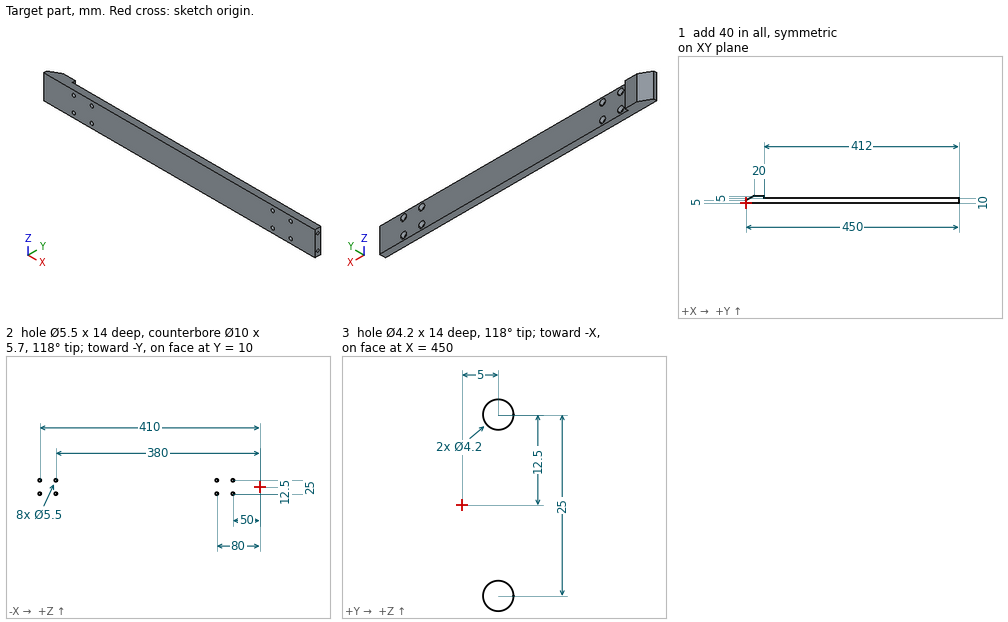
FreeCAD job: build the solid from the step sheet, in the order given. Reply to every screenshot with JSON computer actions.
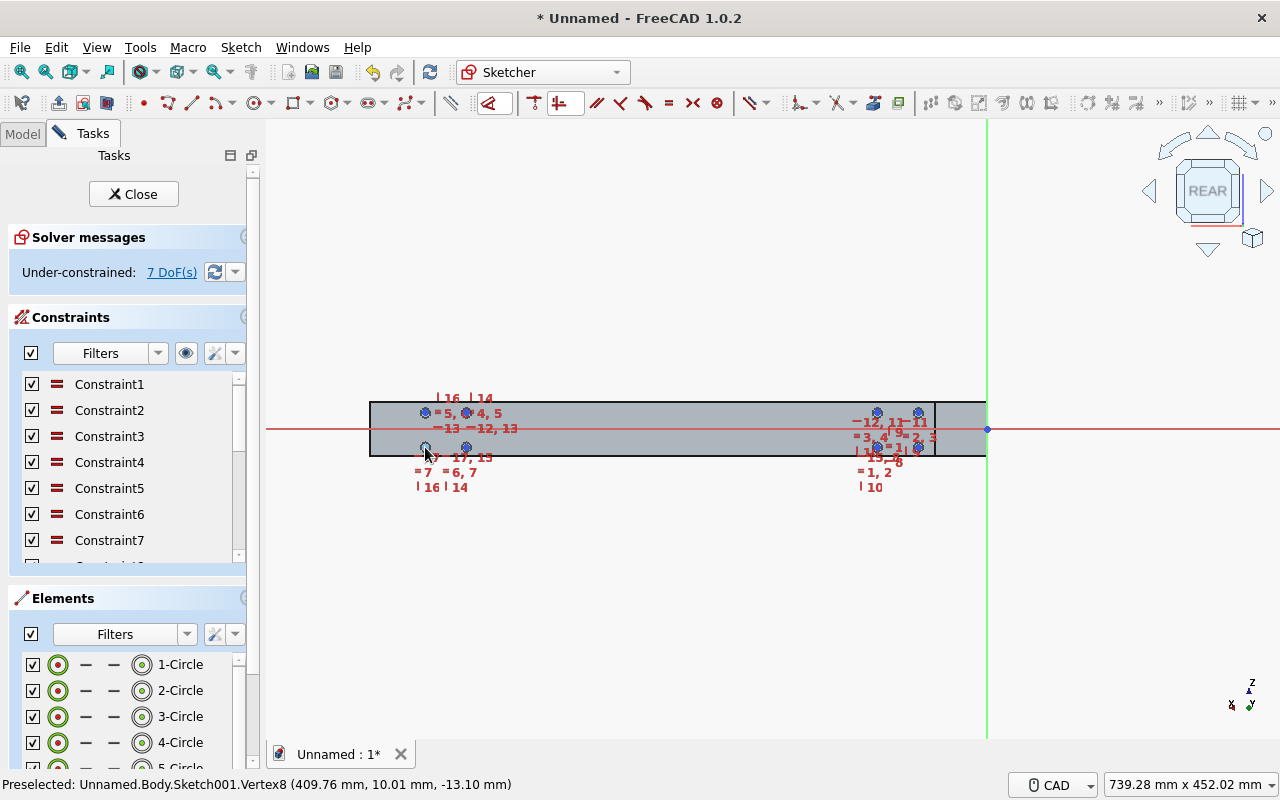
{"action": "scroll", "coordinate": [922, 444], "scroll_direction": "up", "scroll_amount": 9}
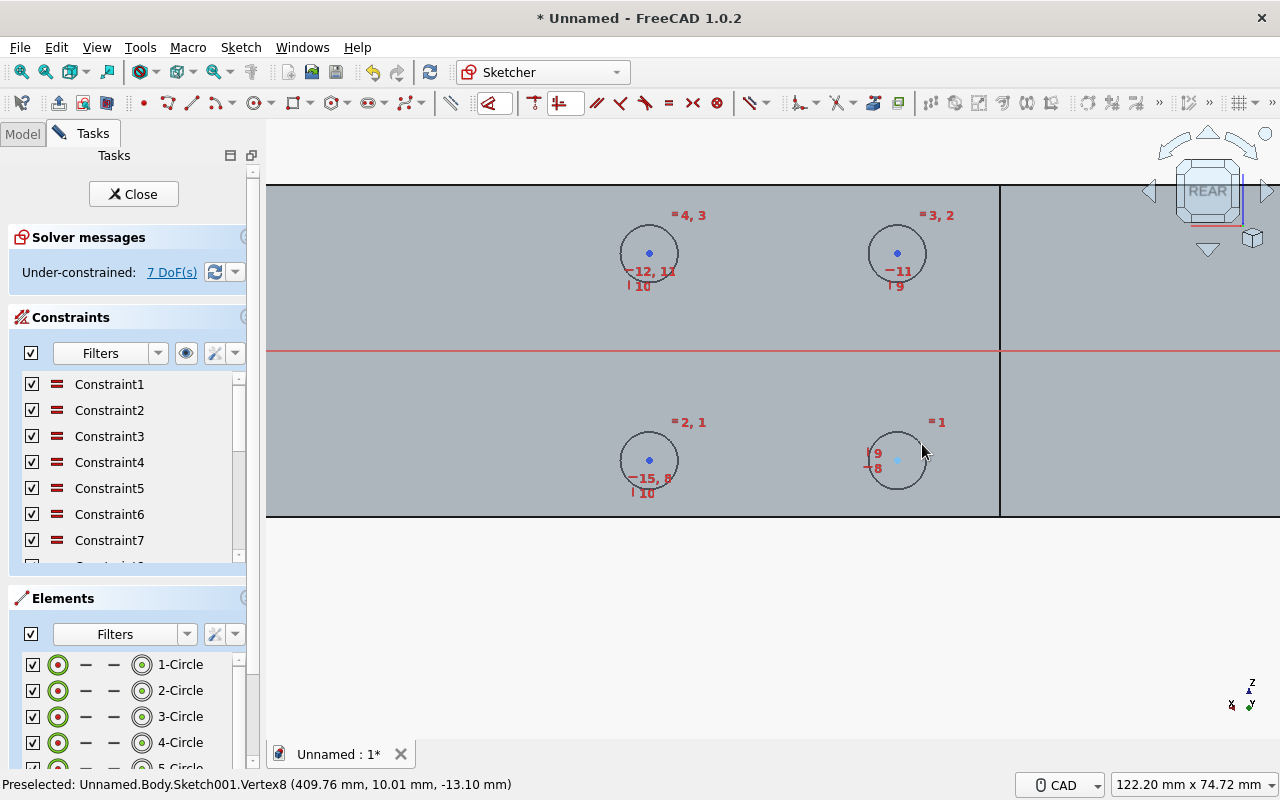
{"action": "left_click", "coordinate": [917, 440]}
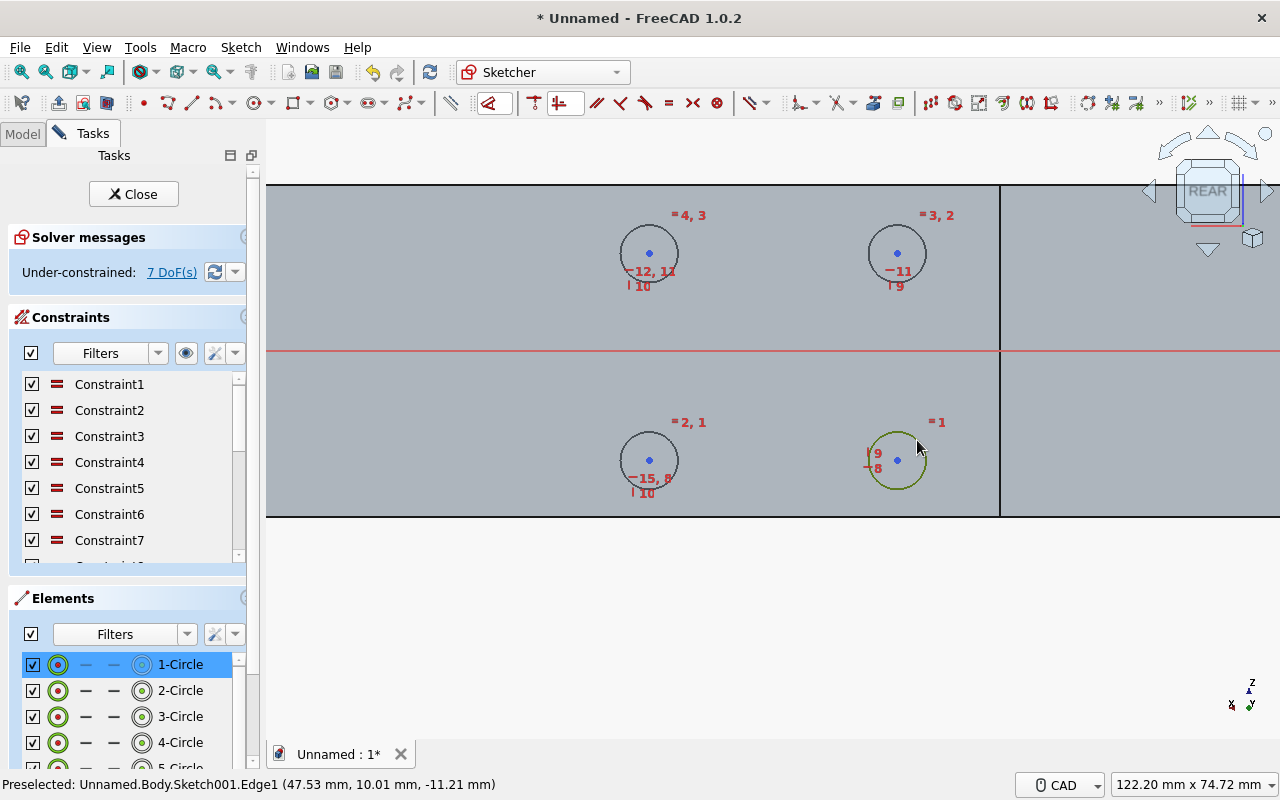
{"action": "left_click", "coordinate": [506, 104]}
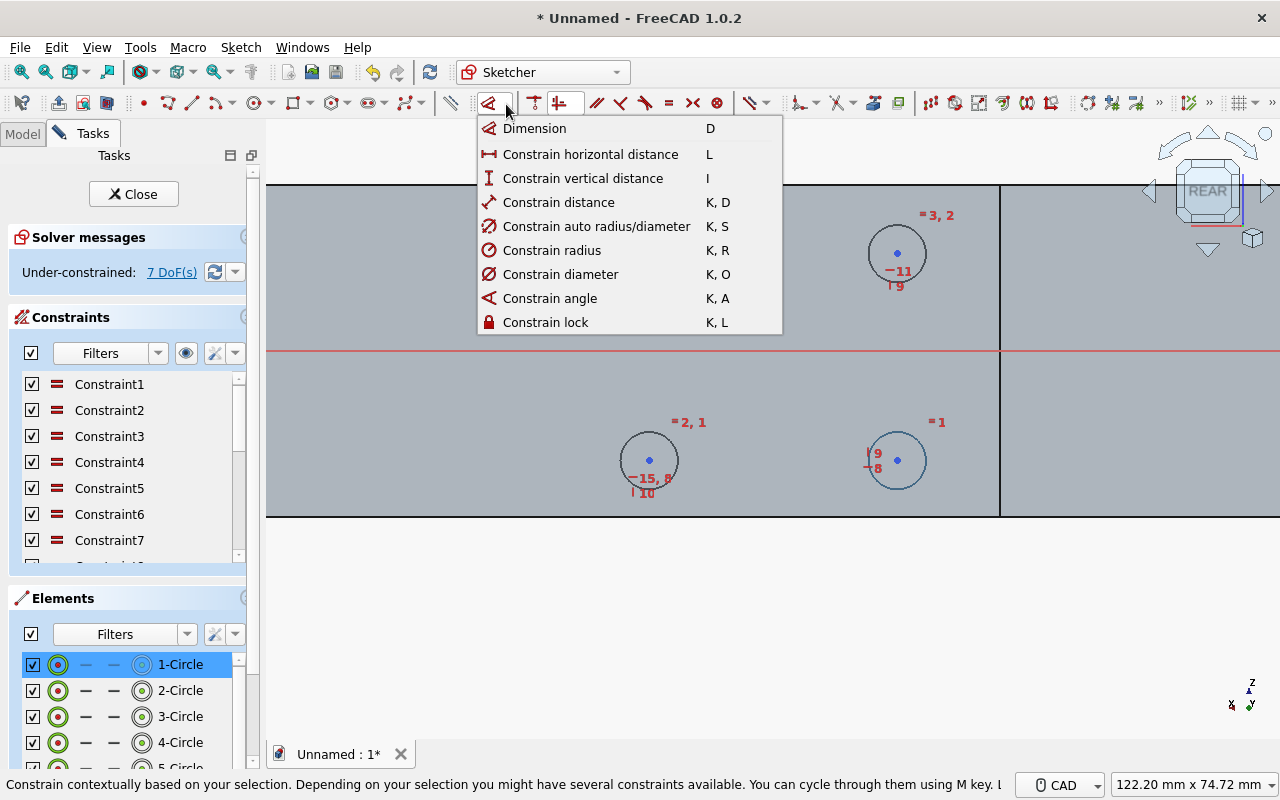
{"action": "left_click", "coordinate": [630, 274]}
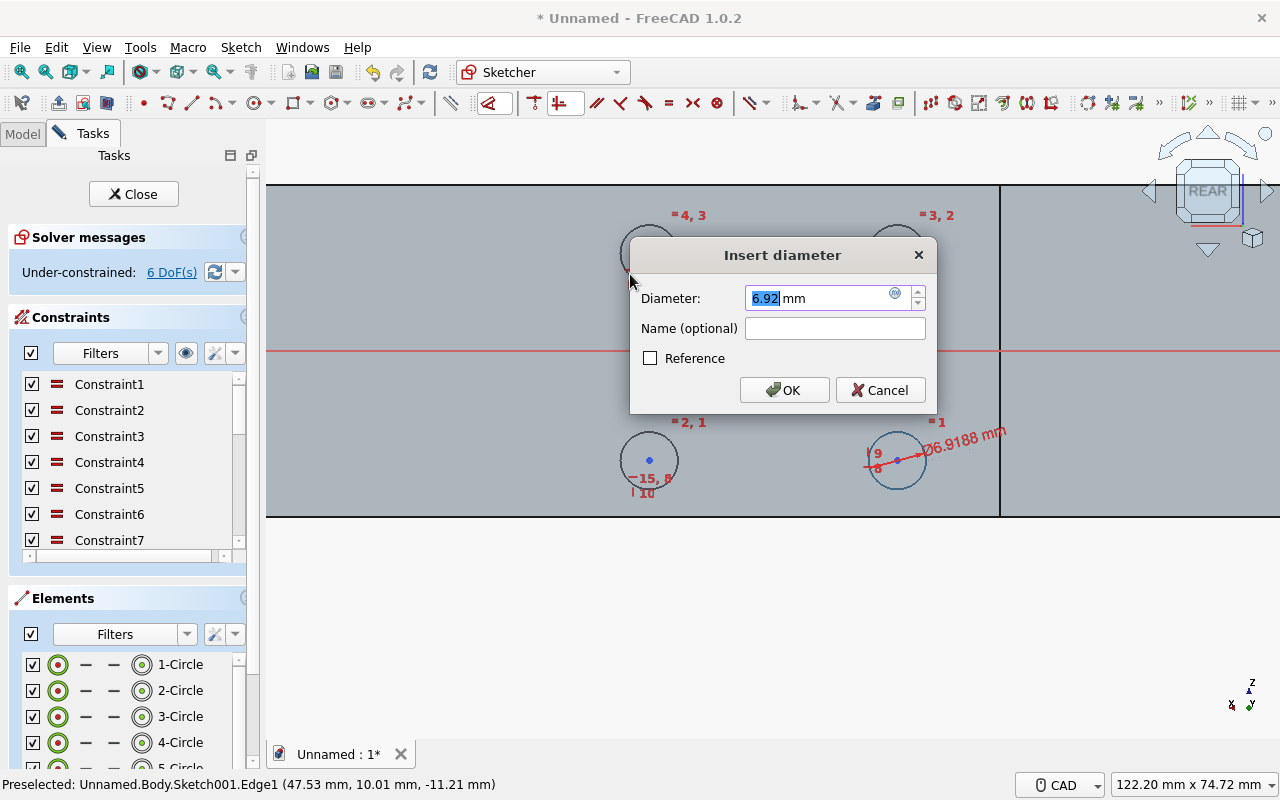
{"action": "type", "text": "5.5"}
{"action": "key", "text": "Return"}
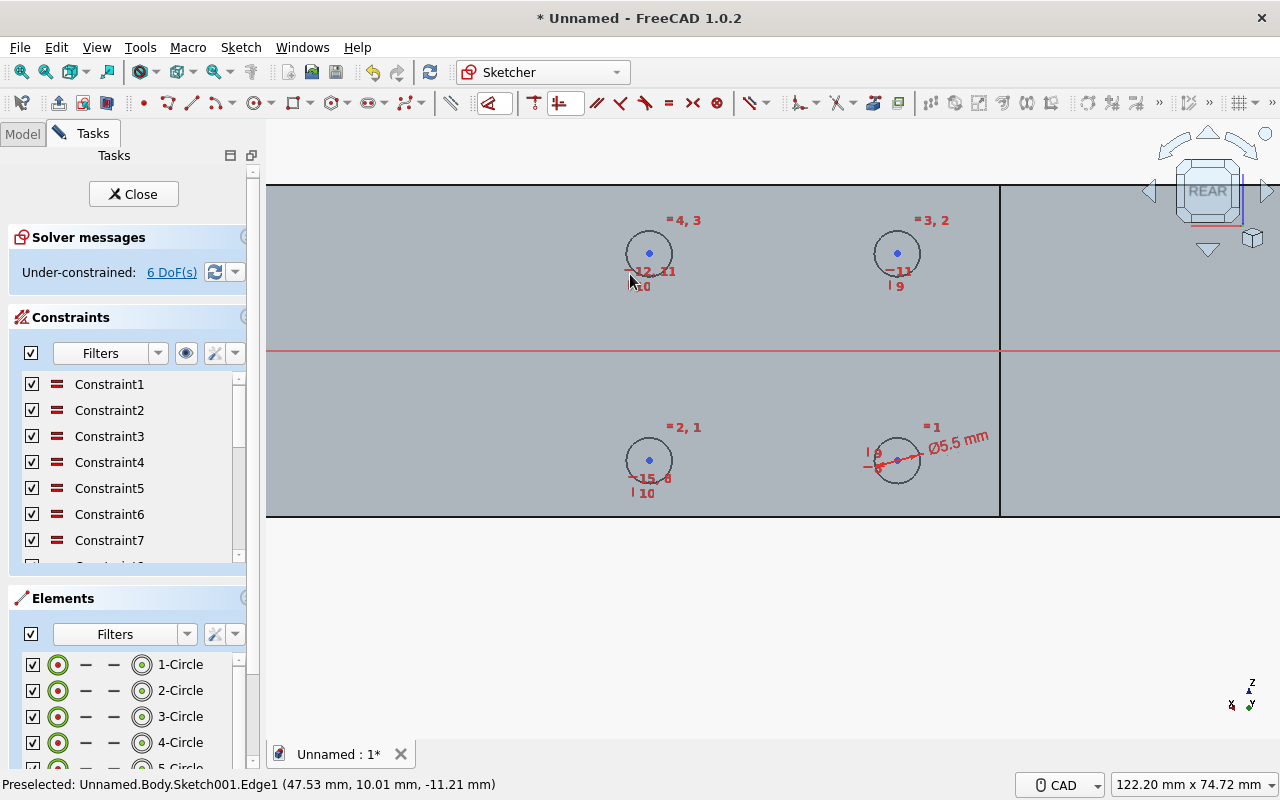
{"action": "scroll", "coordinate": [923, 444], "scroll_direction": "down", "scroll_amount": 9}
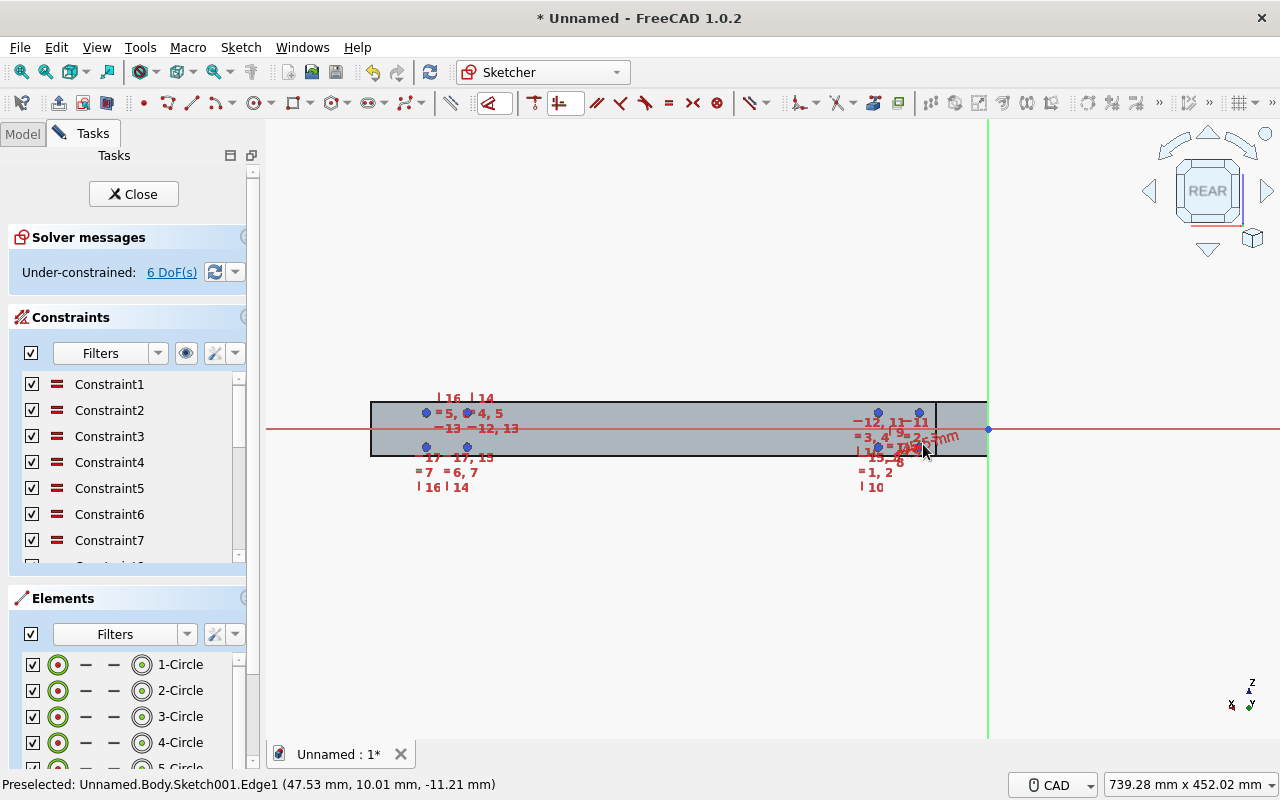
{"action": "left_click", "coordinate": [919, 447]}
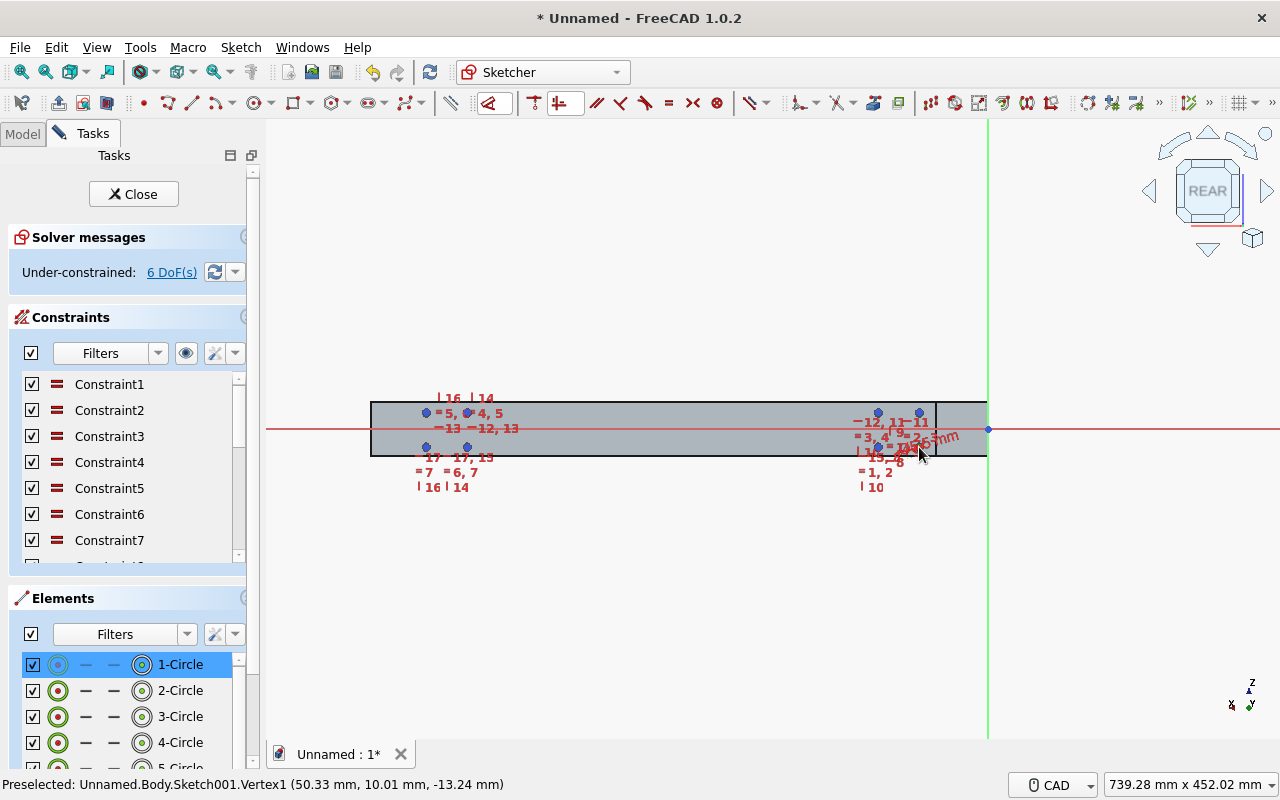
{"action": "key", "text": "l"}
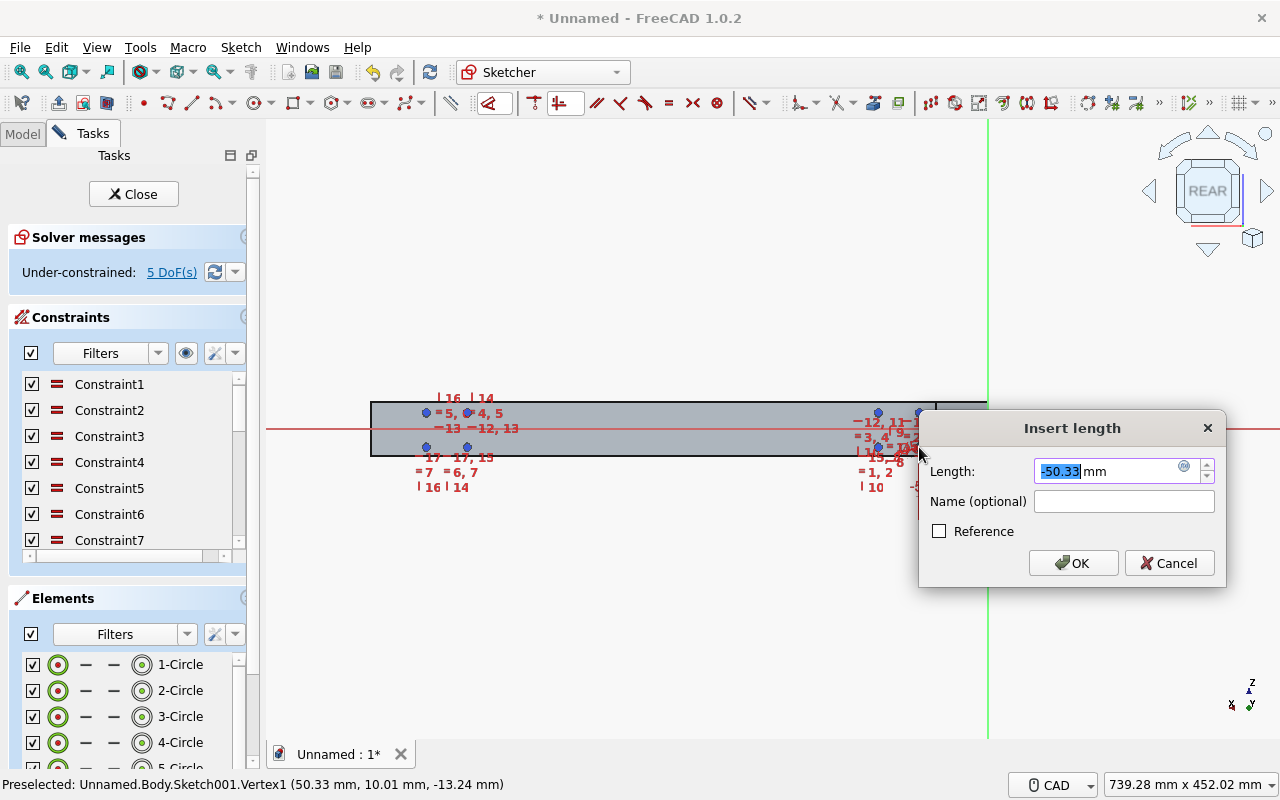
{"action": "type", "text": "-50"}
{"action": "key", "text": "Return"}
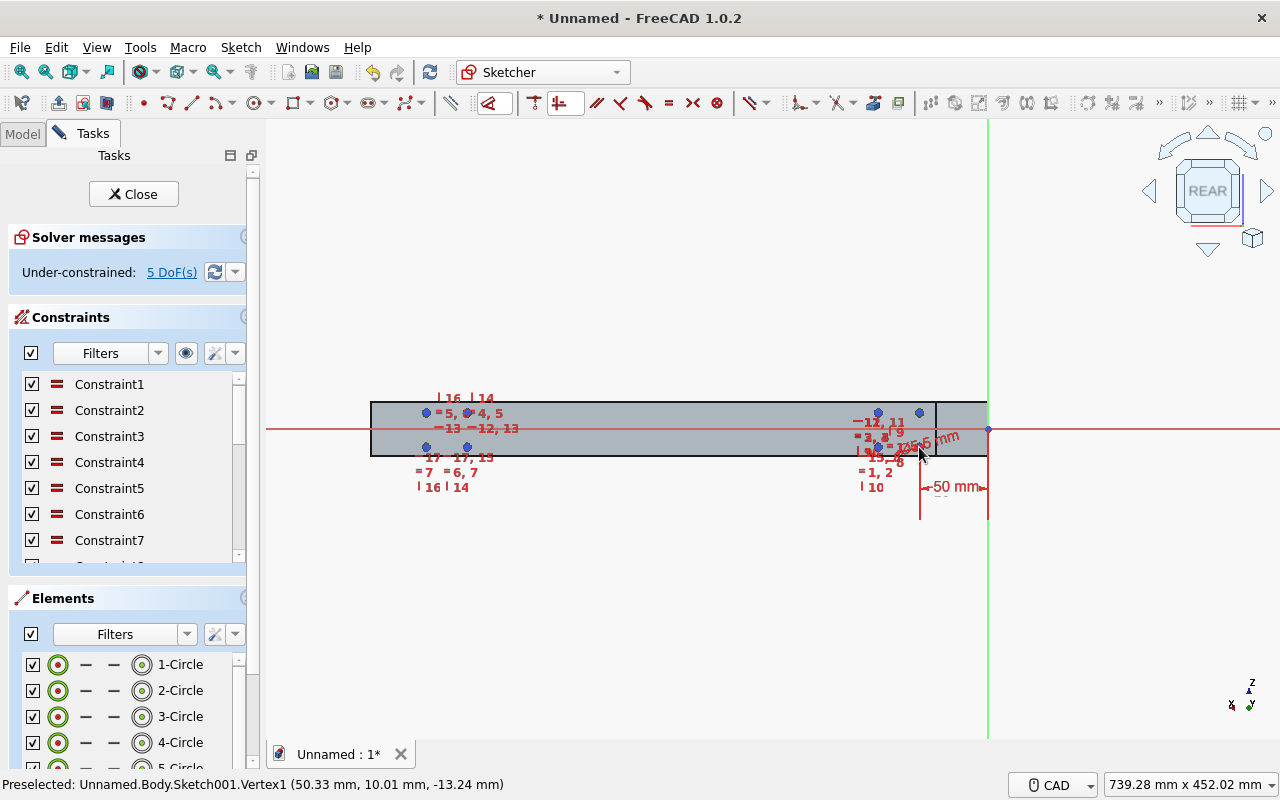
{"action": "left_click", "coordinate": [878, 447]}